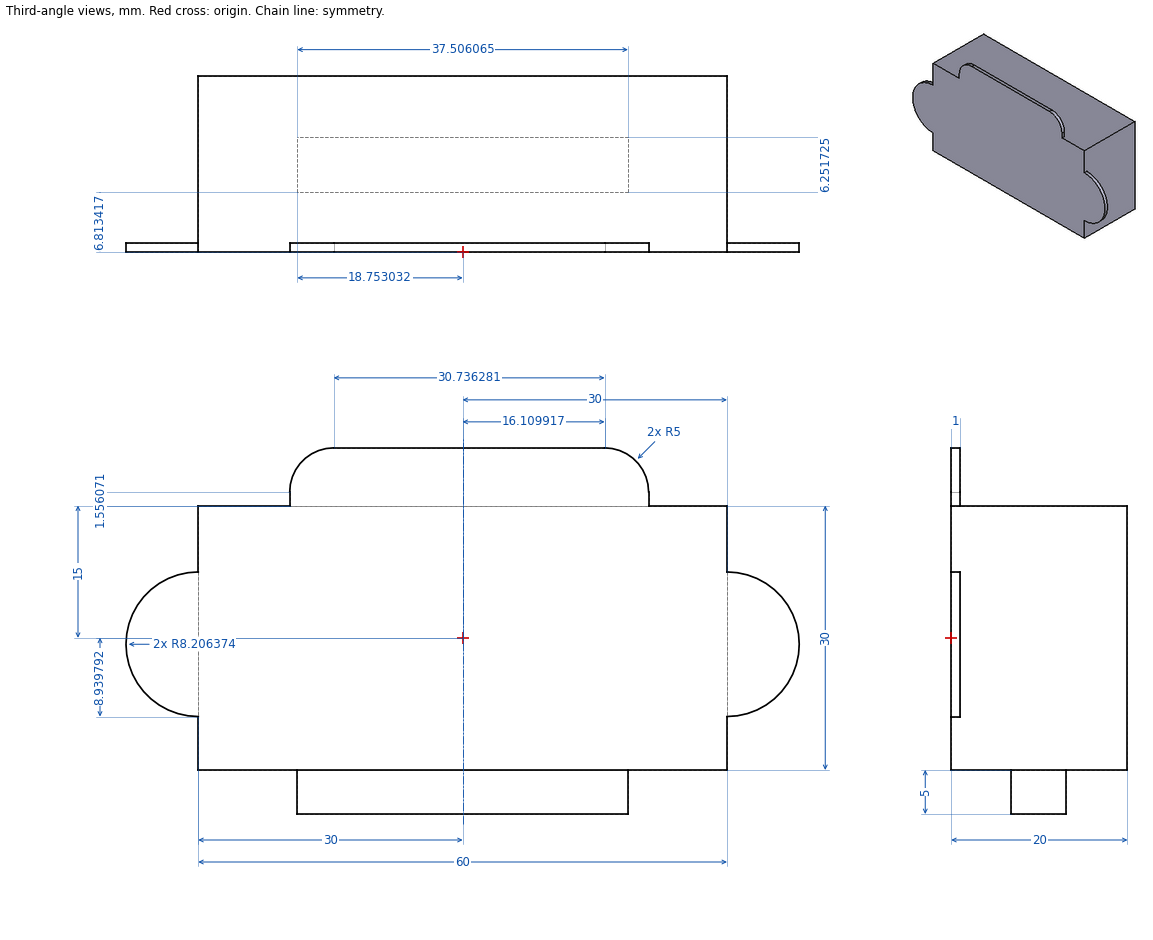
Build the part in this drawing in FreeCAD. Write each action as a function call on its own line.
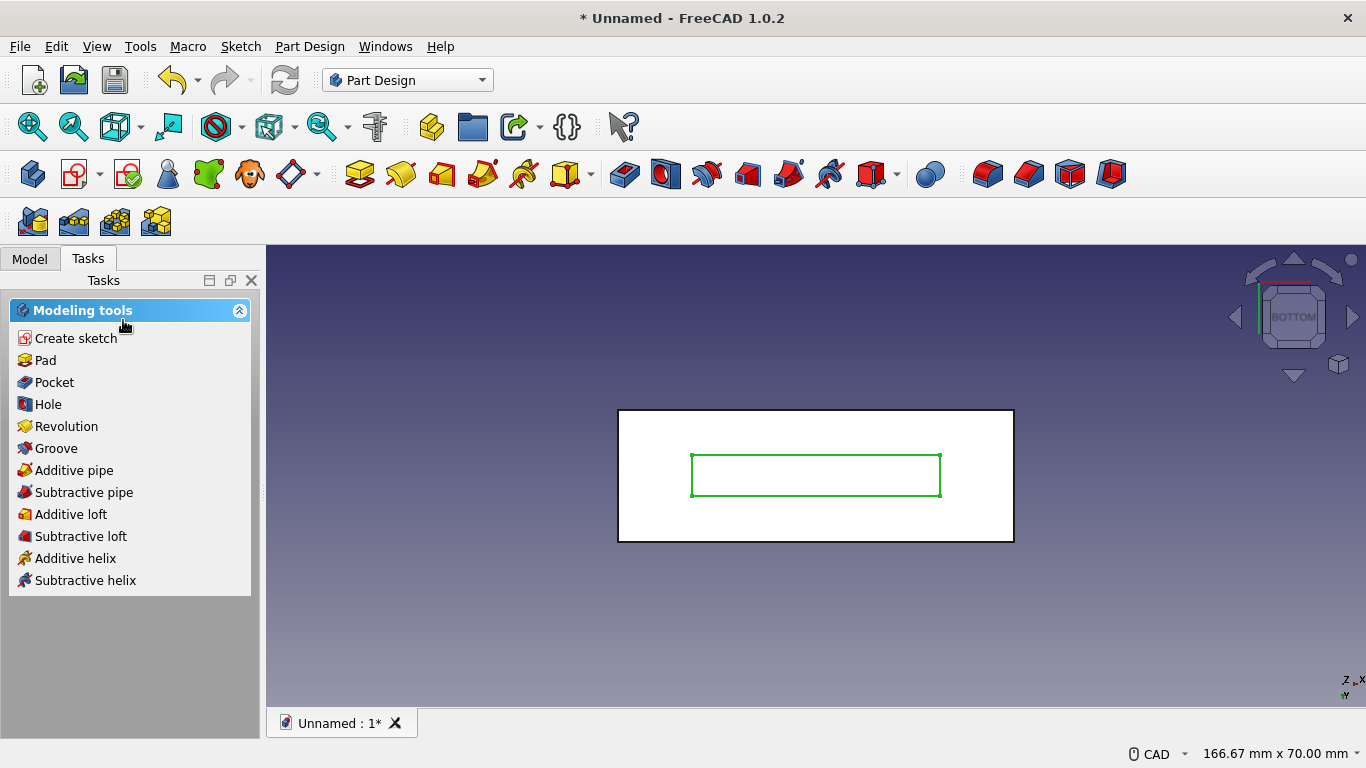
click(360, 174)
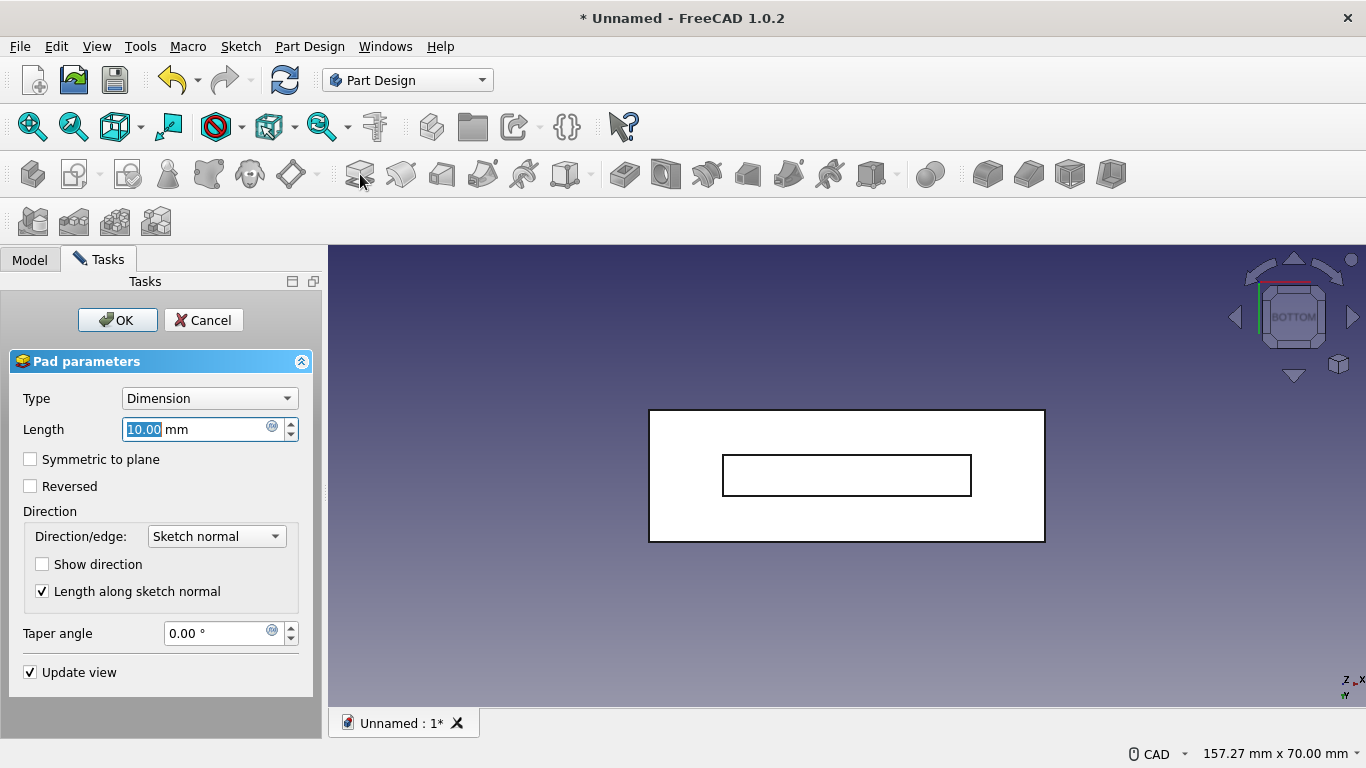
text(5)
key(Tab)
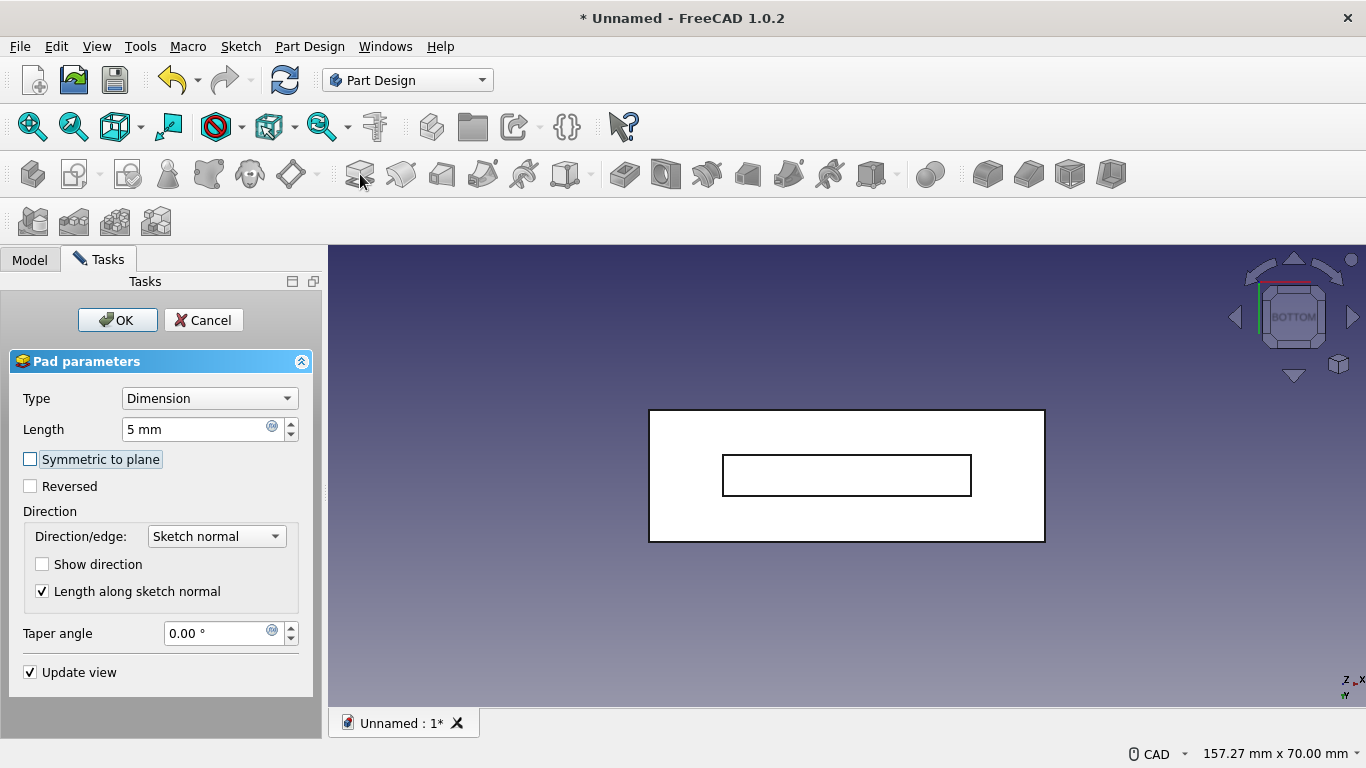
click(118, 320)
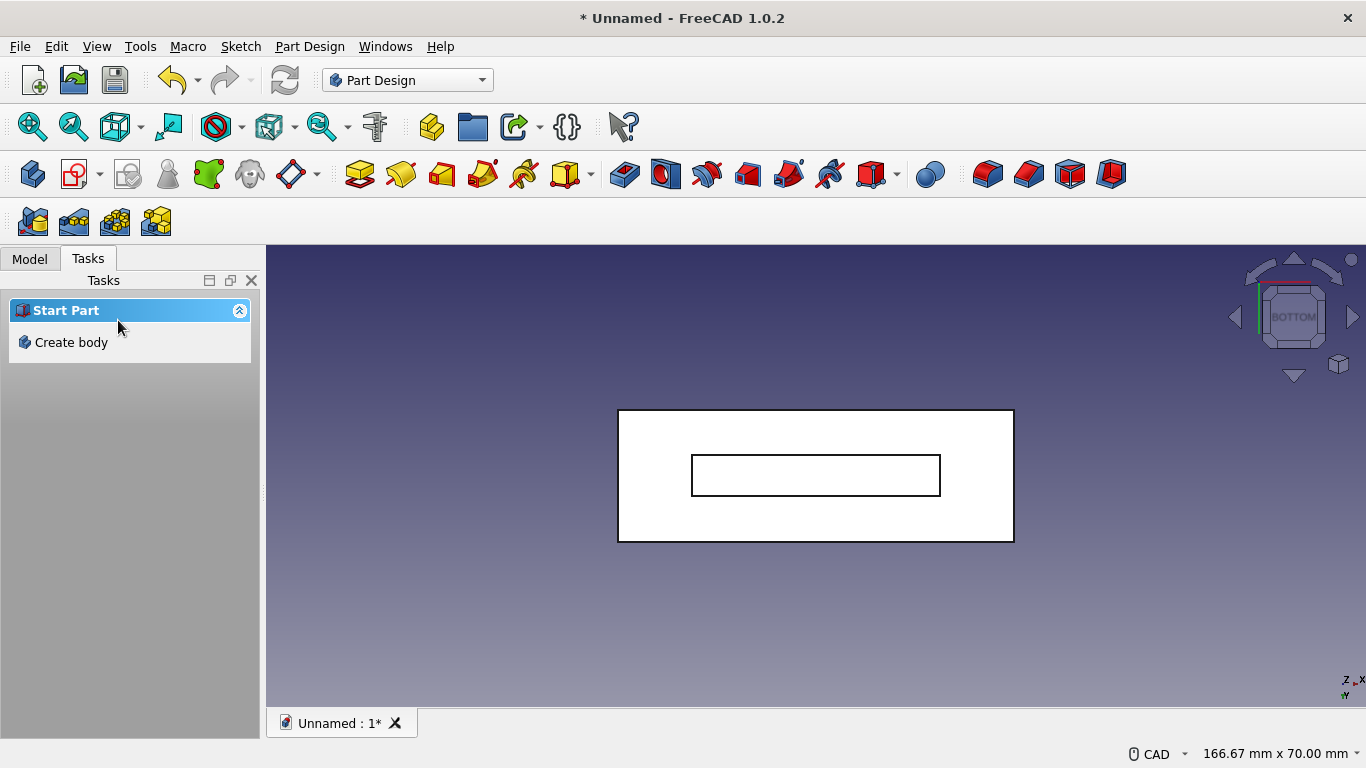
key(v)
key(f)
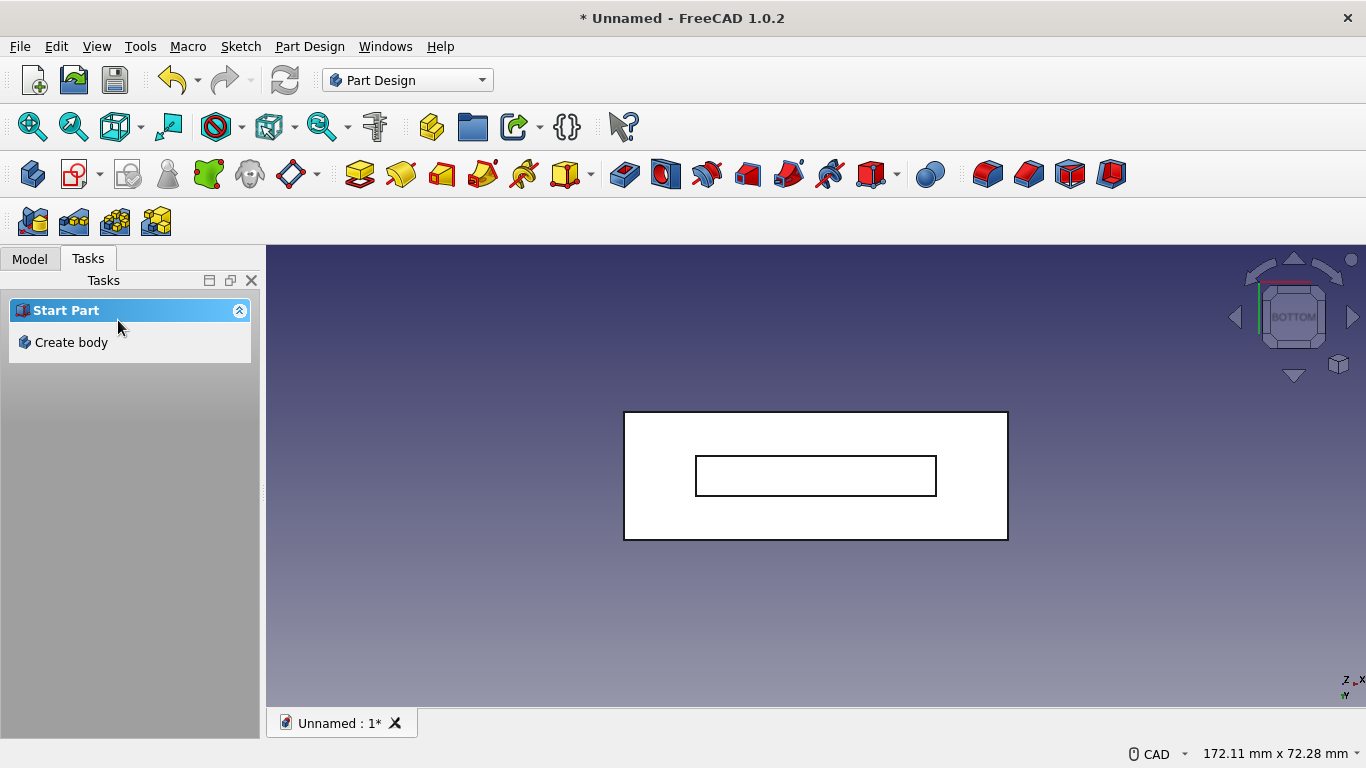
click(74, 174)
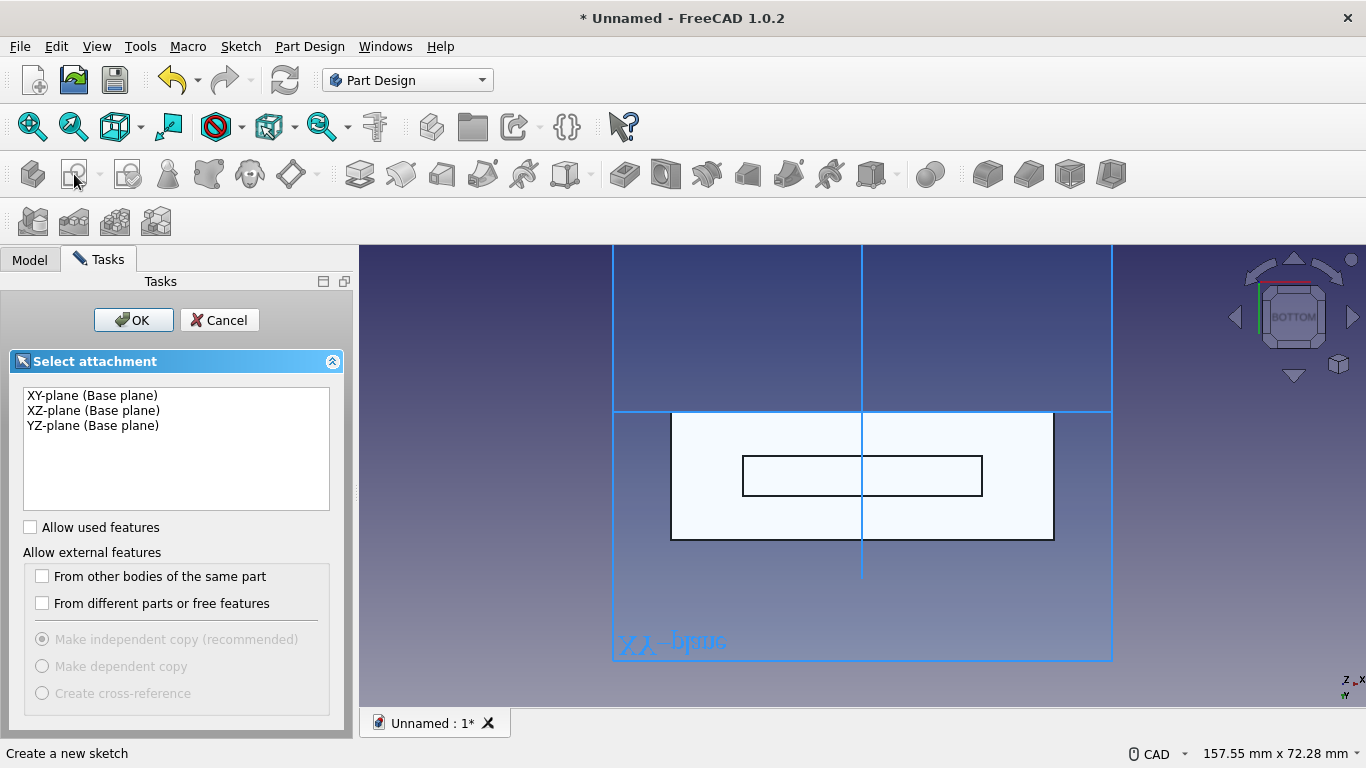
click(84, 410)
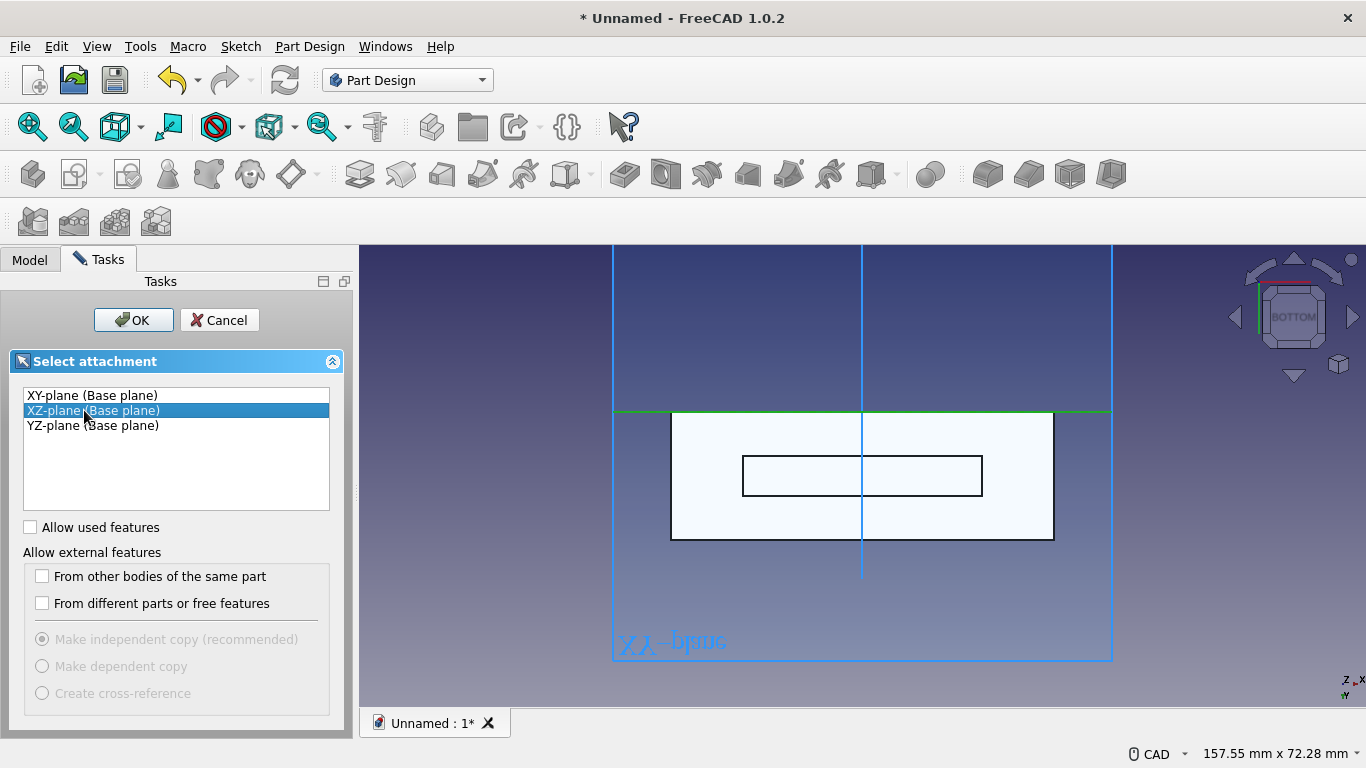
click(134, 320)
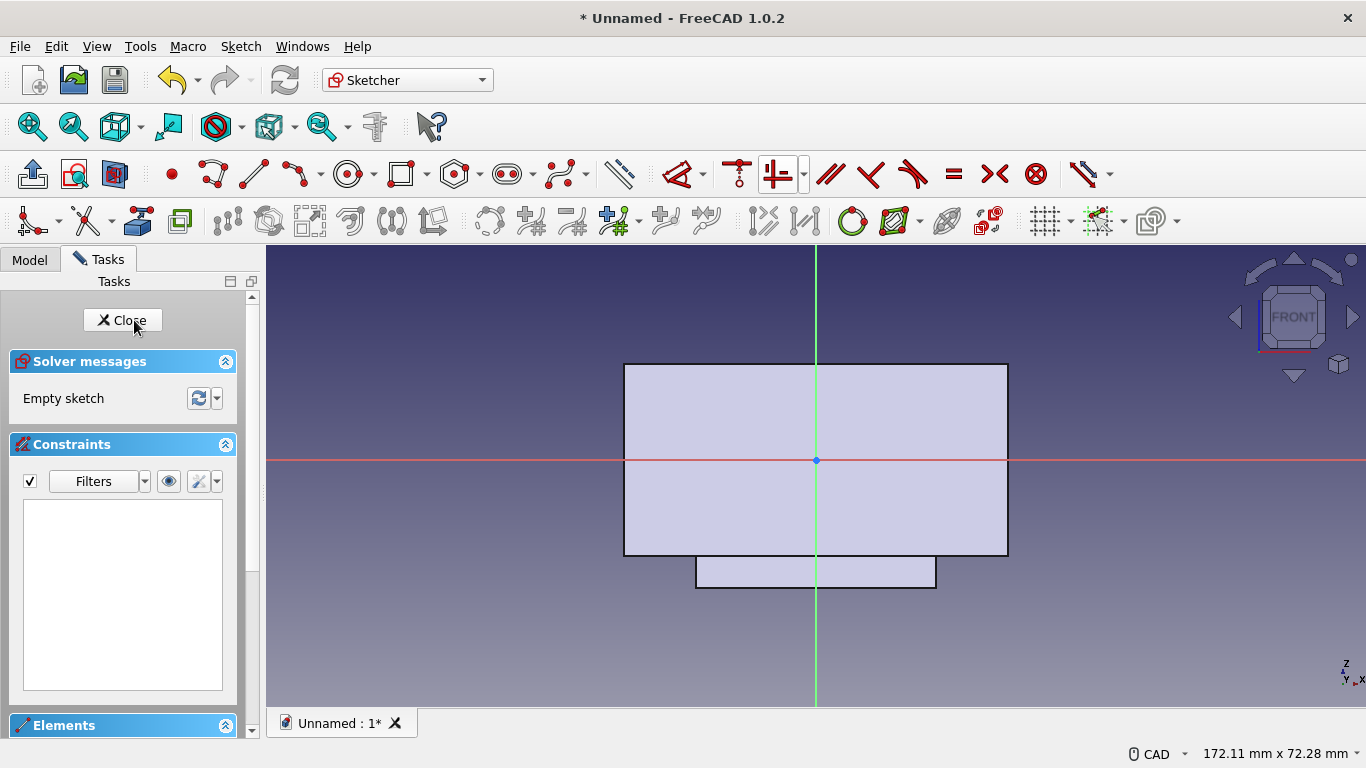
key(g)
key(l)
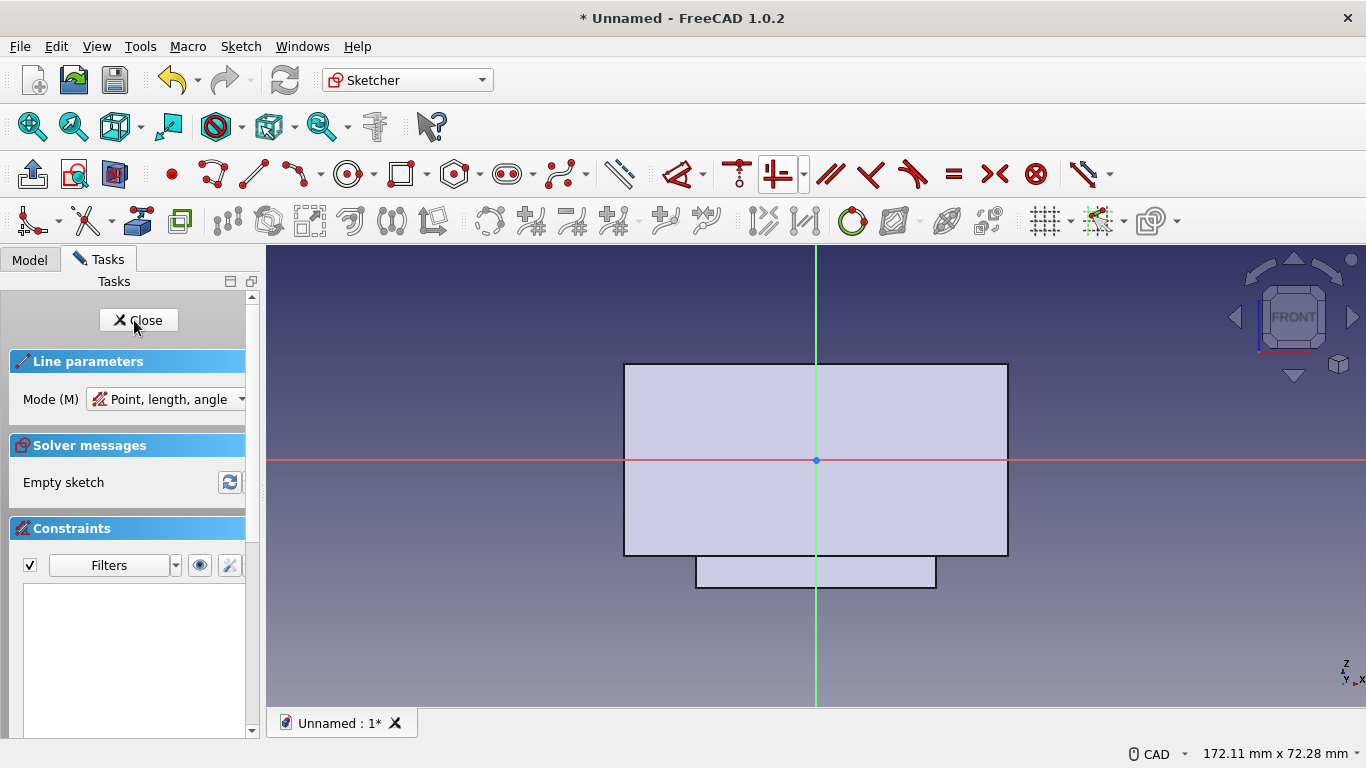
click(624, 517)
click(624, 412)